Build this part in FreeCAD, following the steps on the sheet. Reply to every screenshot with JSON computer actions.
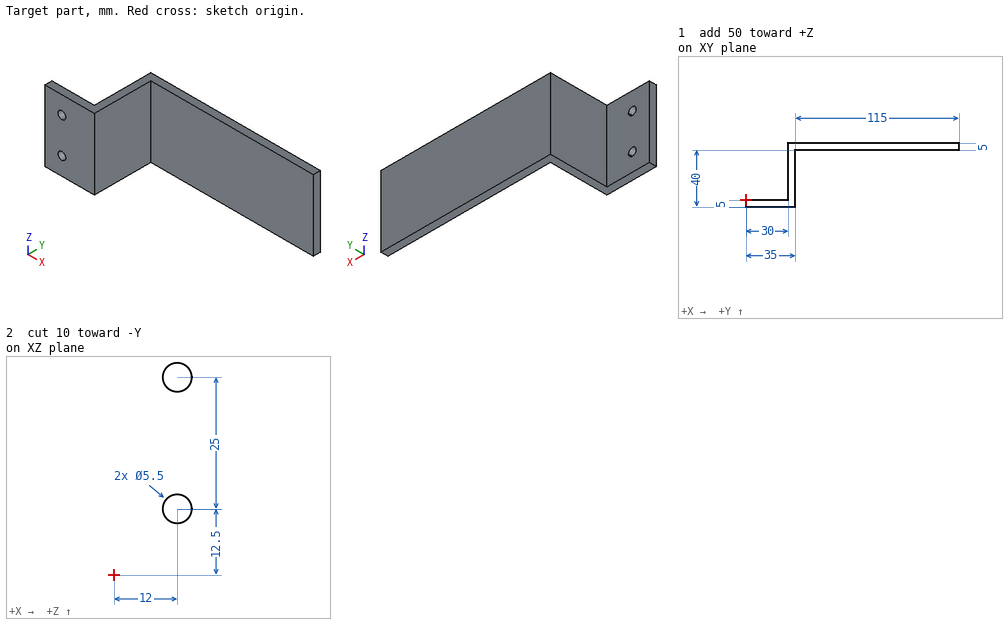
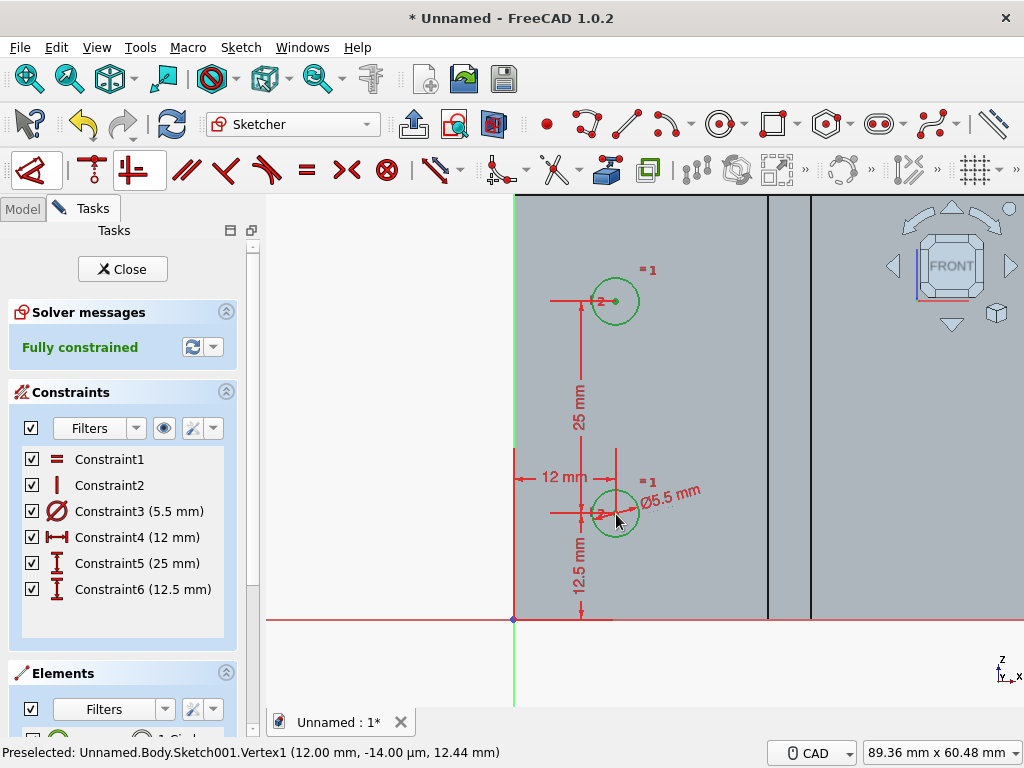
{"action": "left_click", "coordinate": [123, 269]}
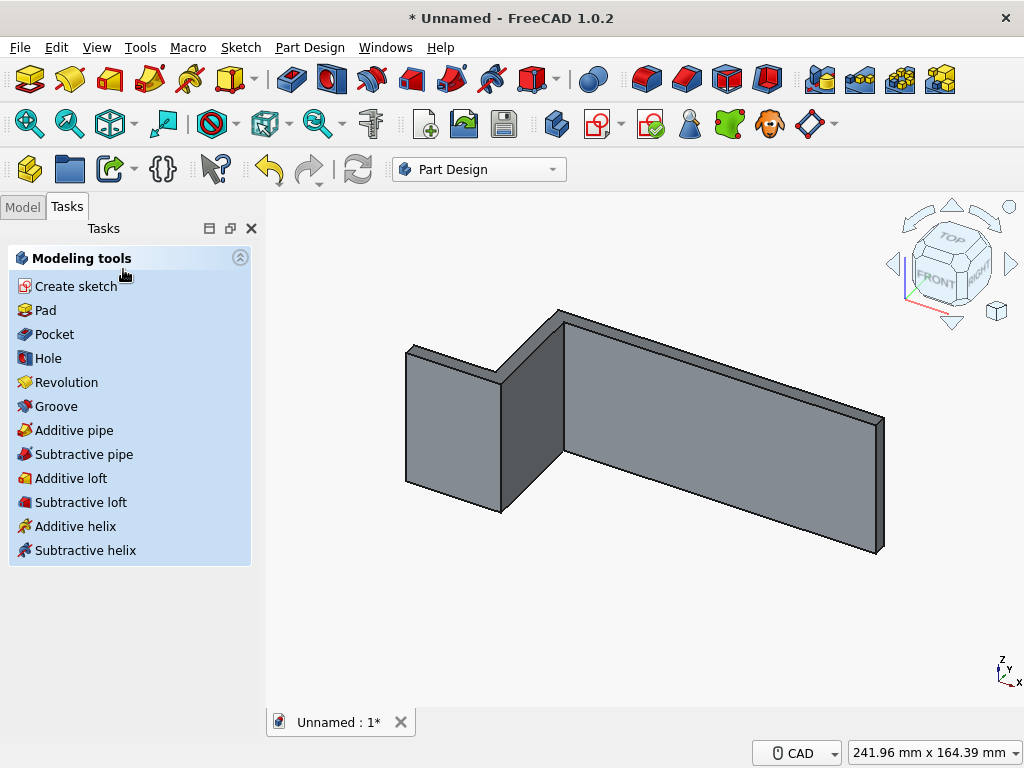
{"action": "left_click", "coordinate": [292, 80]}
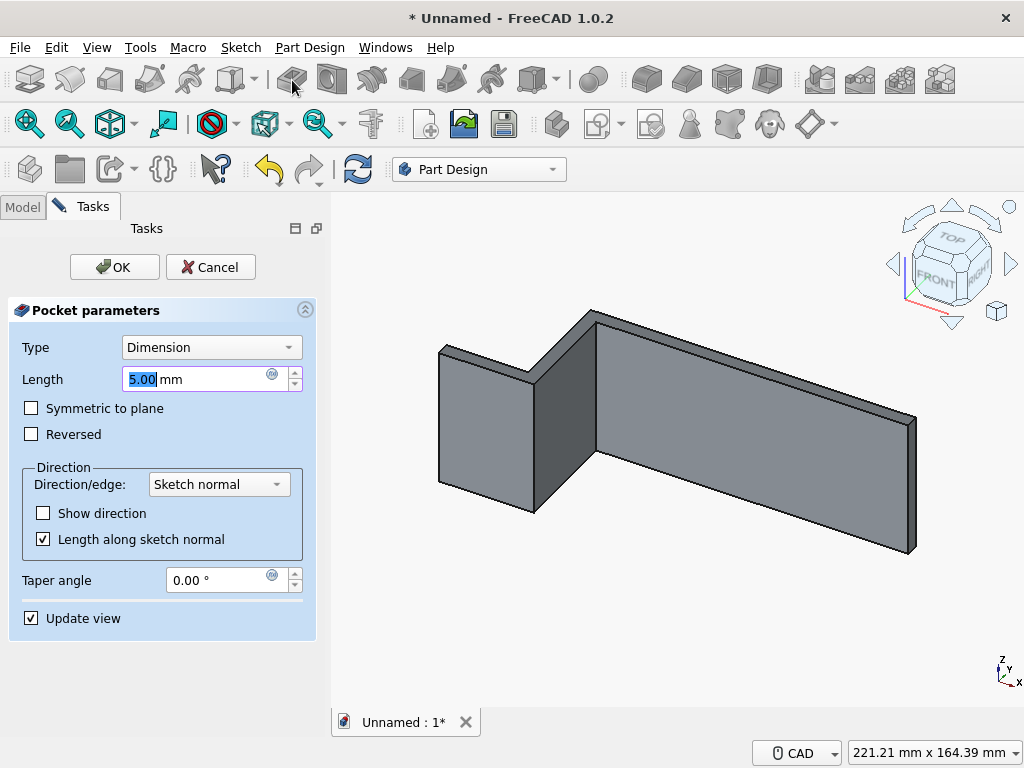
{"action": "type", "text": "10"}
{"action": "key", "text": "Tab"}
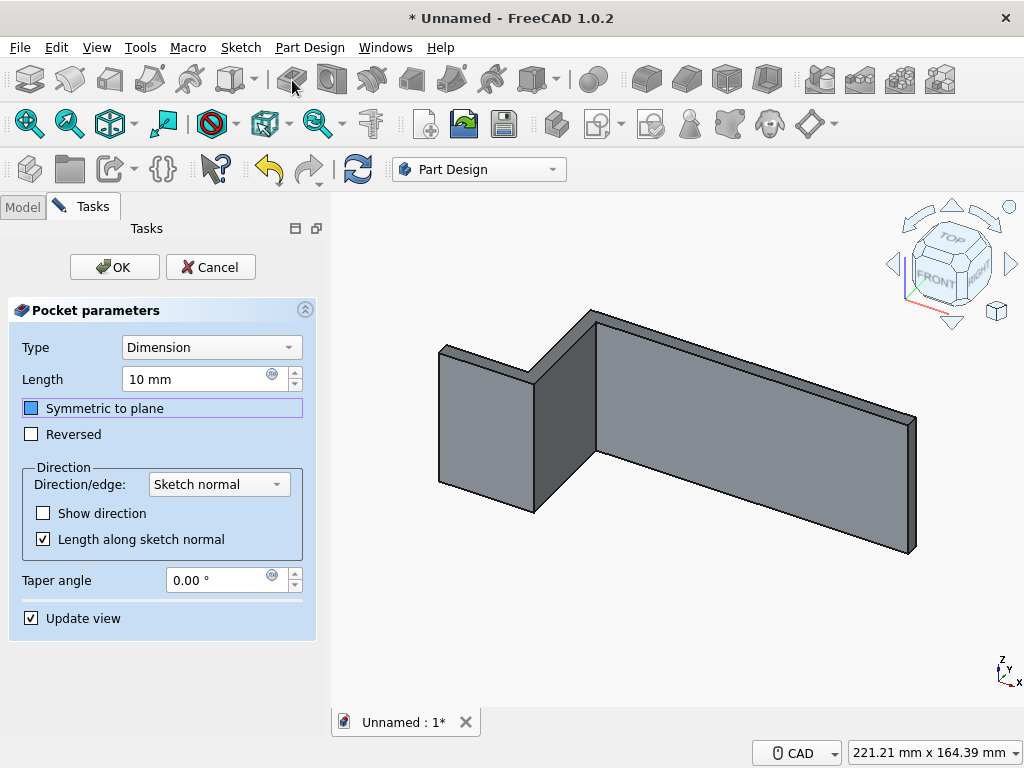
{"action": "left_click", "coordinate": [30, 434]}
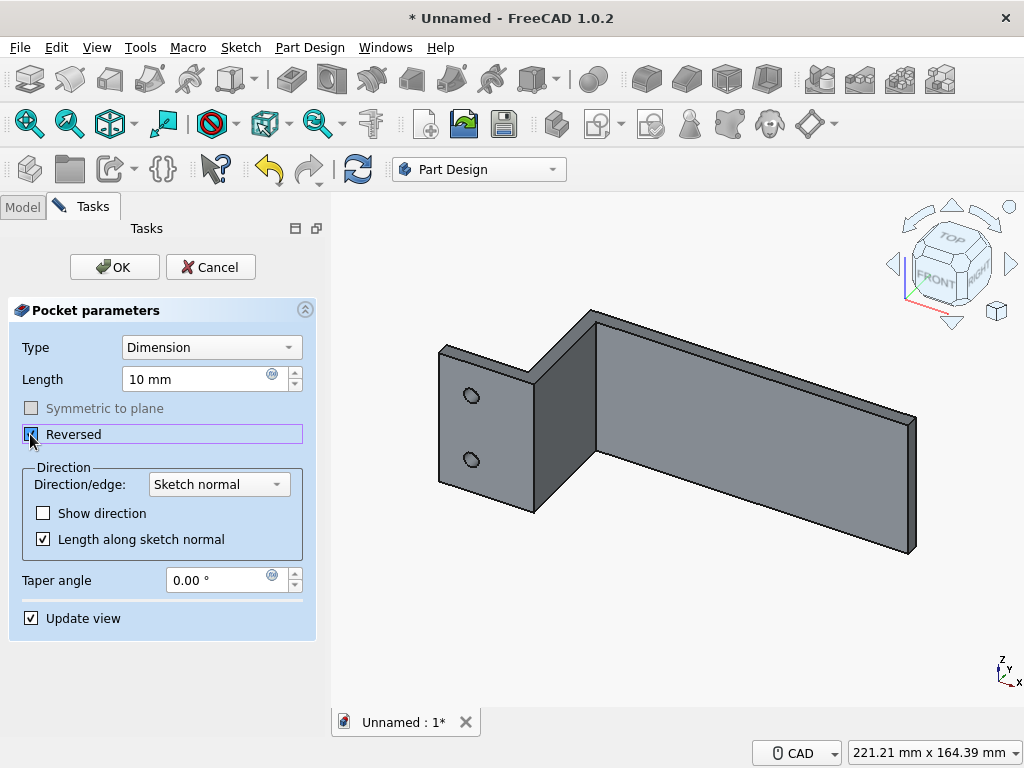
{"action": "left_click", "coordinate": [115, 267]}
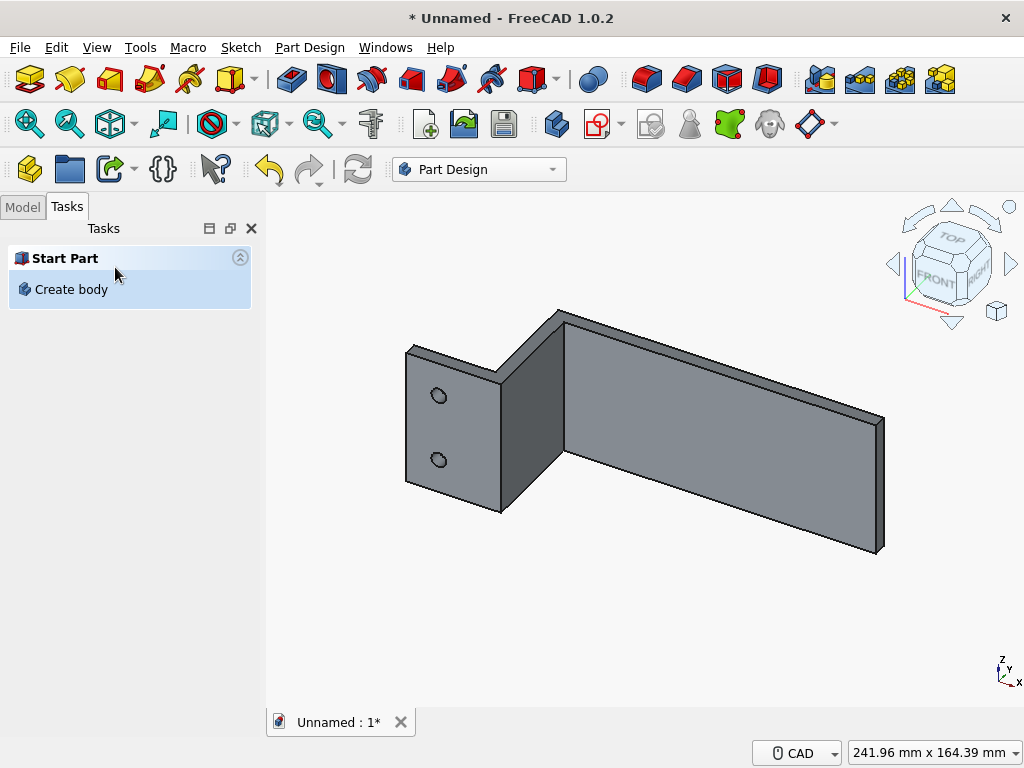
{"action": "key", "text": "0"}